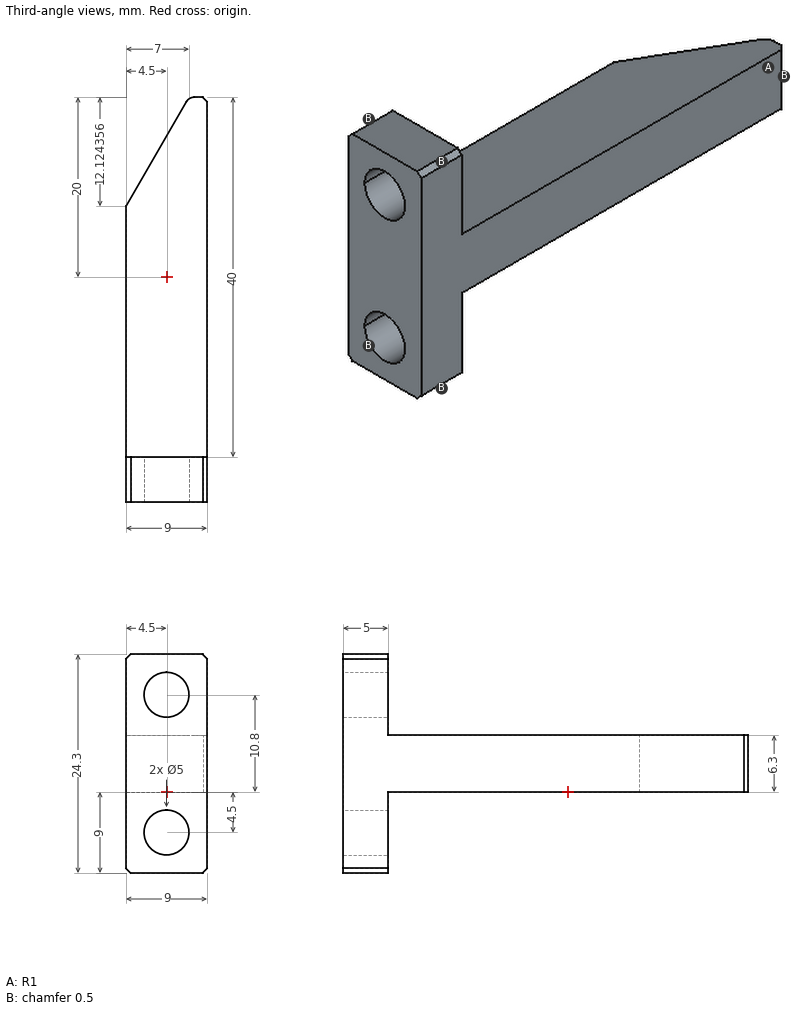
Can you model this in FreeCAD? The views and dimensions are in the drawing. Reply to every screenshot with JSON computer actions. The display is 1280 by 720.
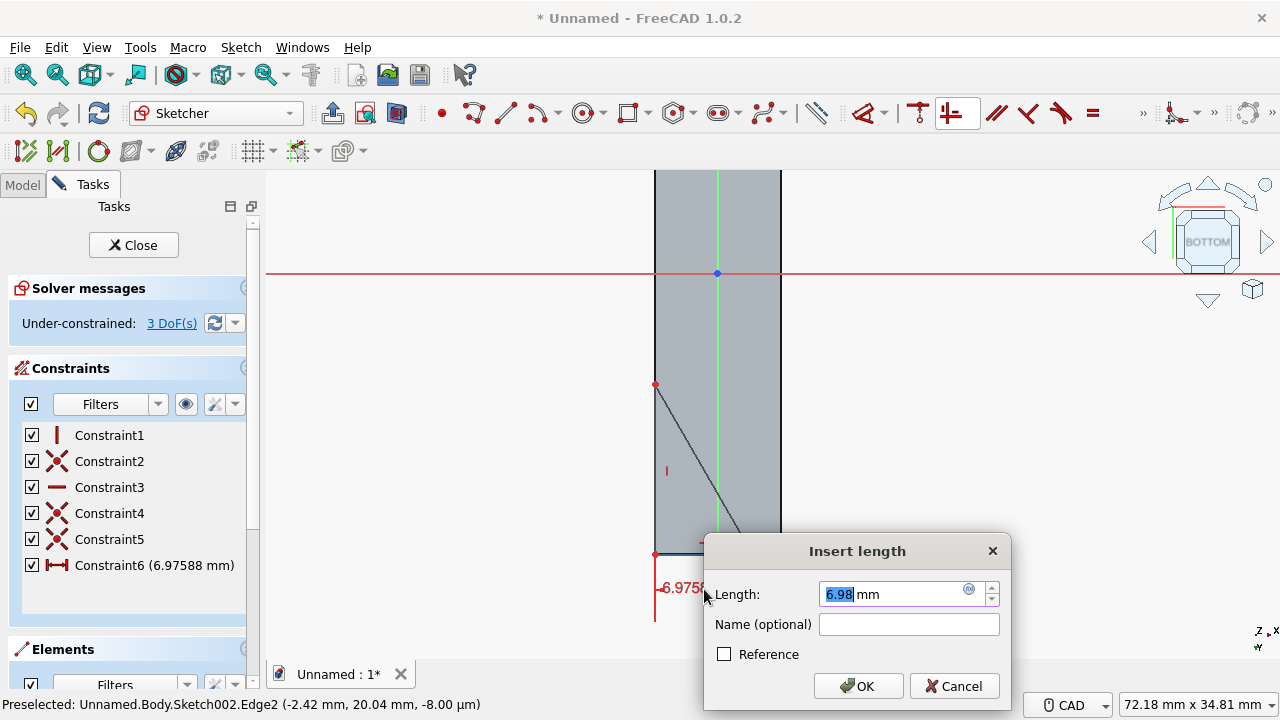
{"action": "type", "text": "7"}
{"action": "key", "text": "Return"}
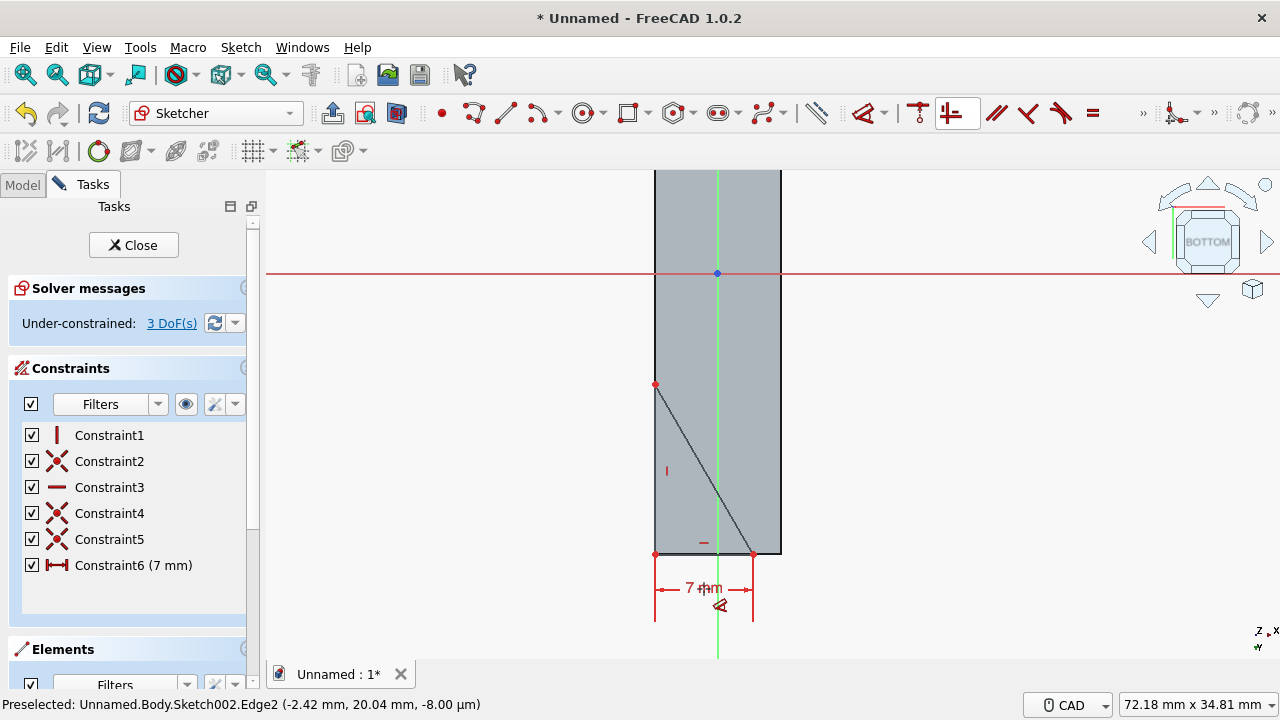
{"action": "left_click", "coordinate": [655, 555]}
{"action": "left_click", "coordinate": [621, 414]}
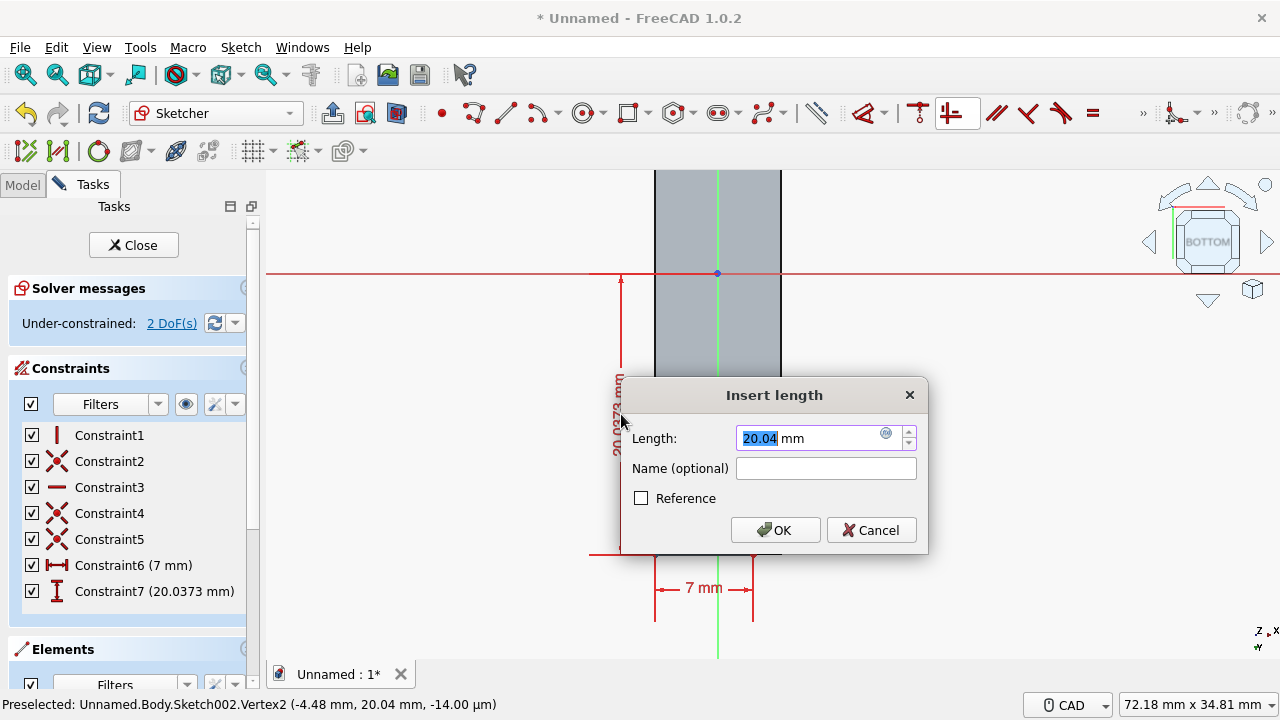
{"action": "type", "text": "20"}
{"action": "key", "text": "Return"}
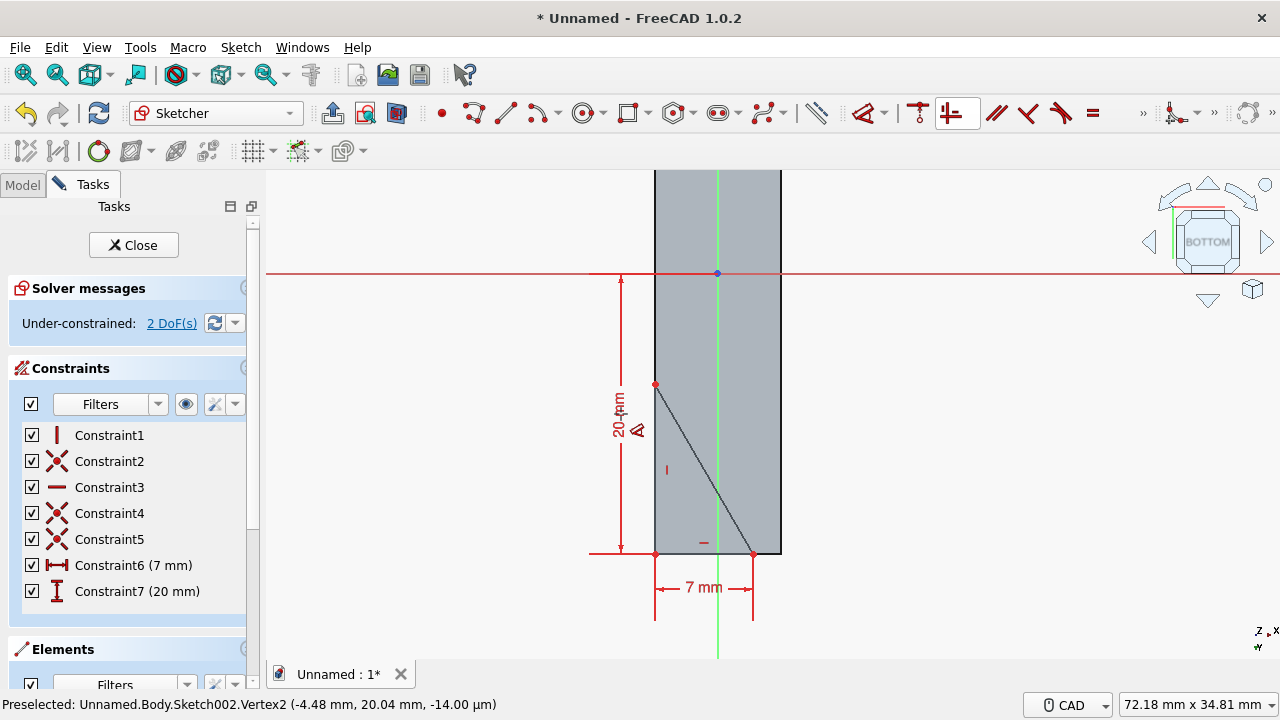
{"action": "left_click", "coordinate": [655, 385]}
{"action": "left_click", "coordinate": [686, 240]}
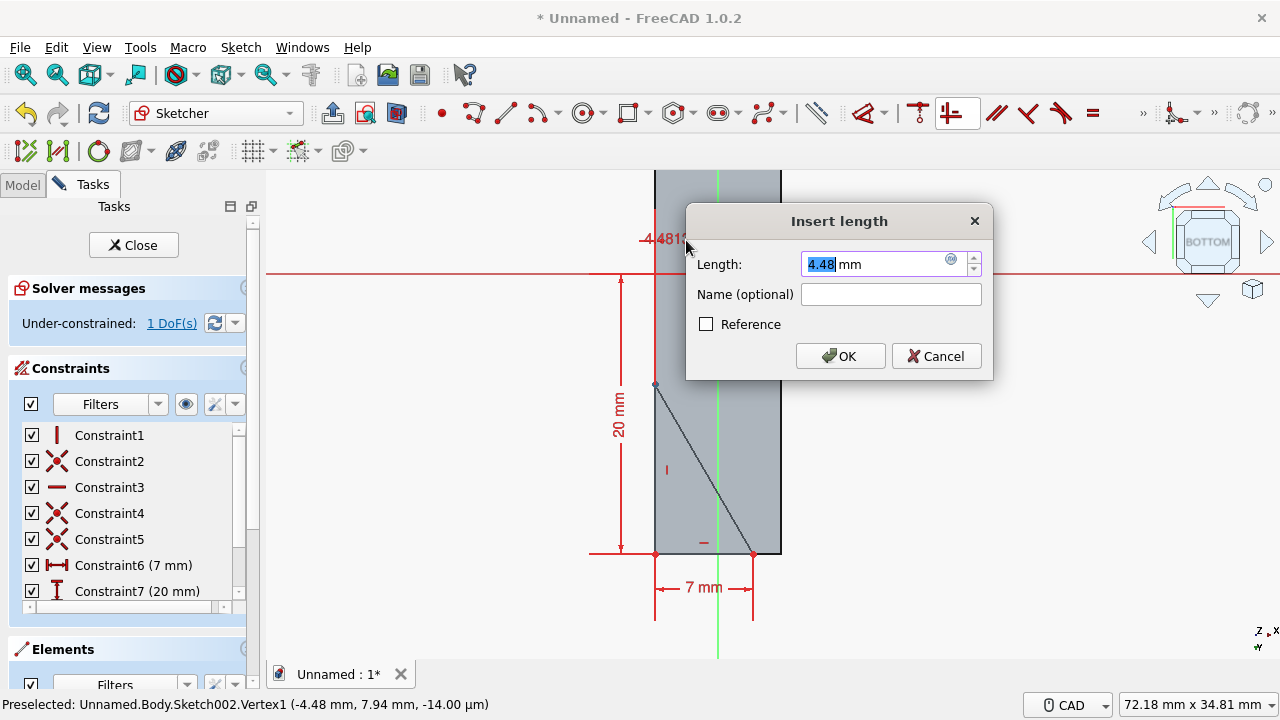
{"action": "type", "text": "4.5"}
{"action": "key", "text": "Return"}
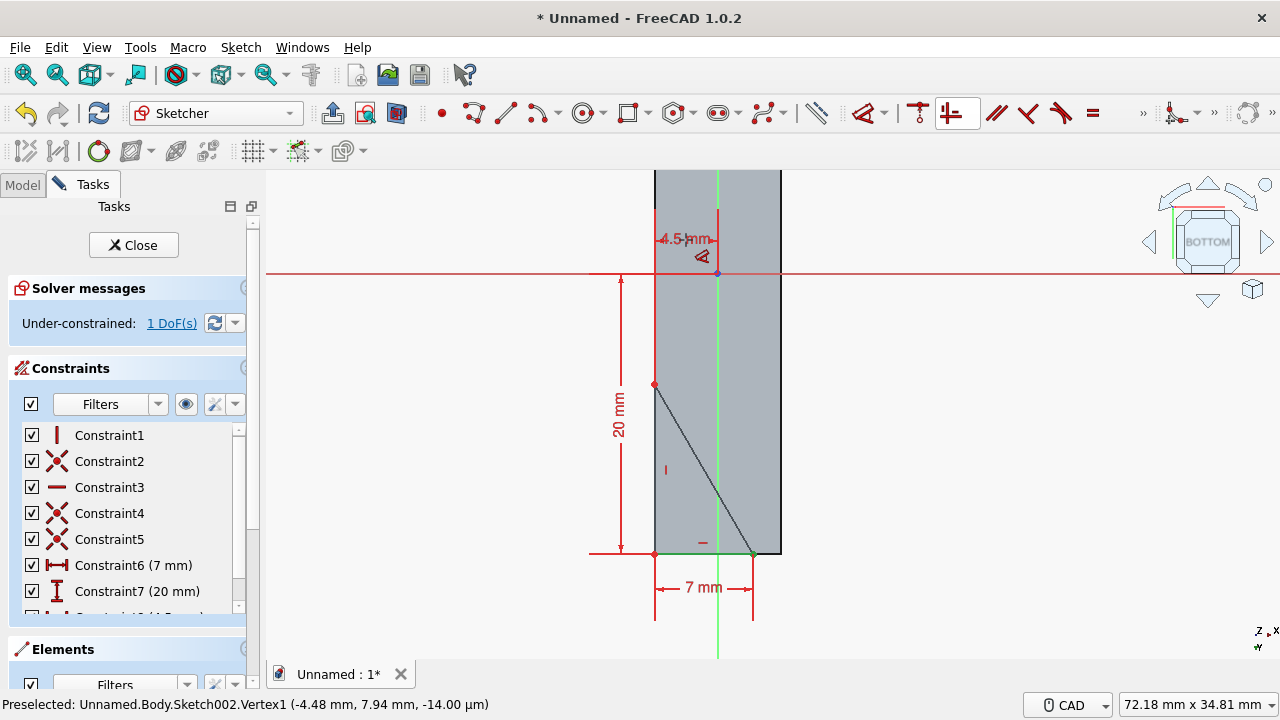
{"action": "left_click", "coordinate": [655, 436]}
{"action": "left_click", "coordinate": [621, 470]}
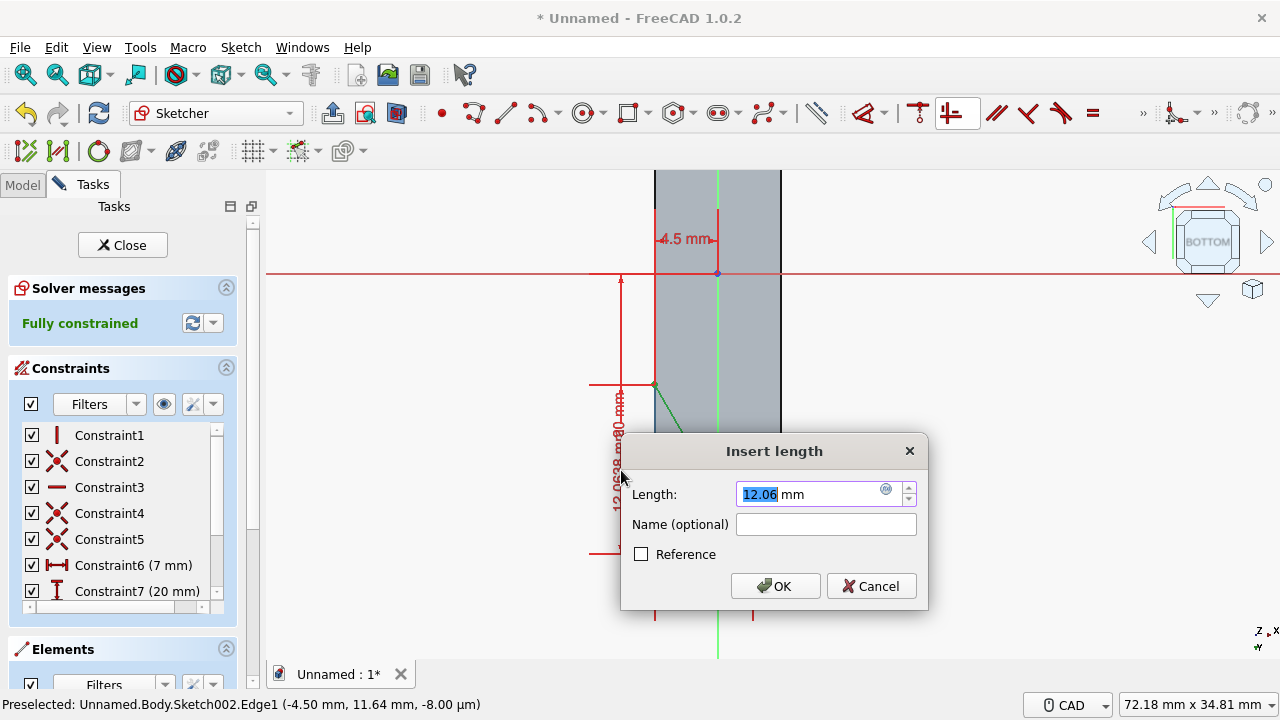
{"action": "type", "text": "12.124356"}
{"action": "key", "text": "Return"}
{"action": "key", "text": "Escape"}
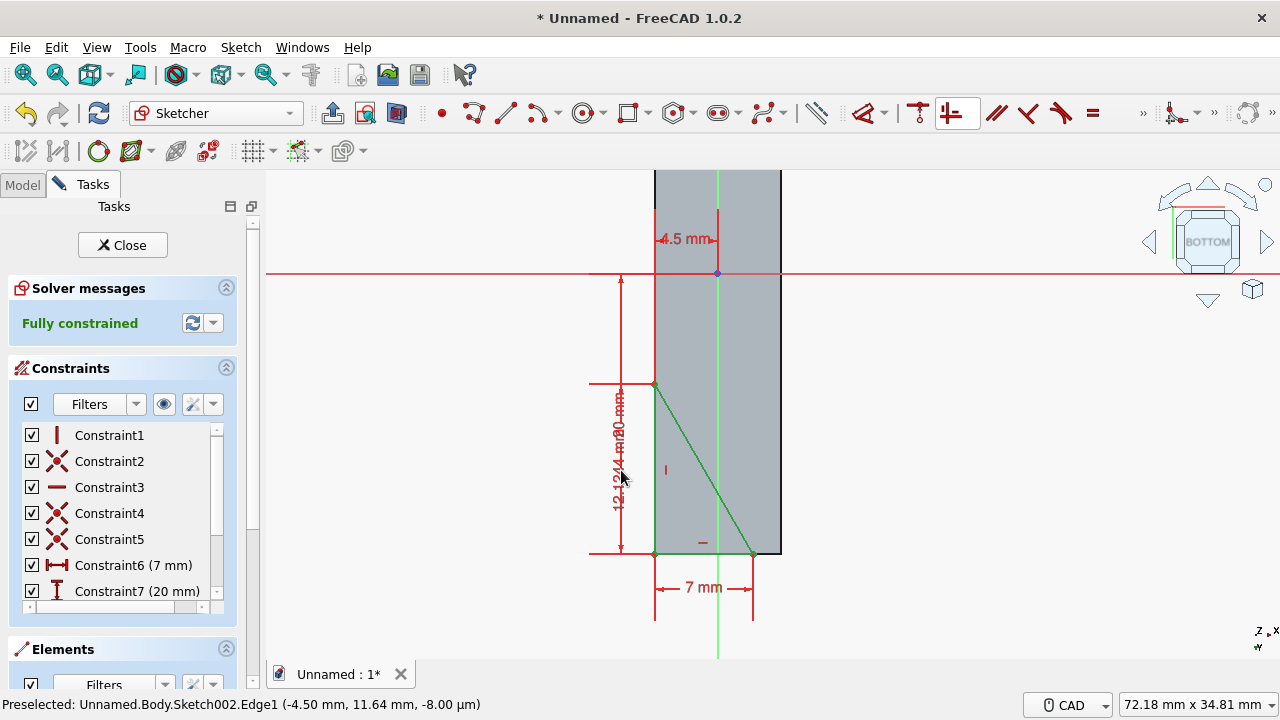
{"action": "left_click", "coordinate": [123, 245]}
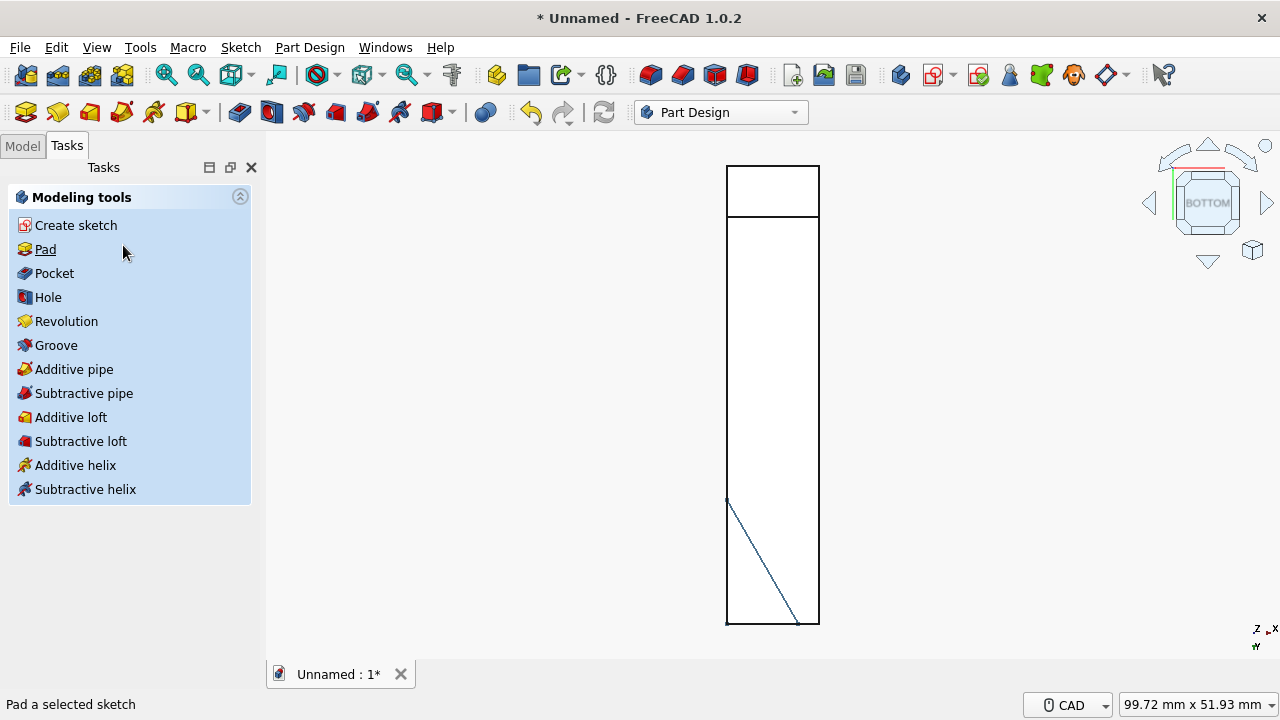
{"action": "left_click", "coordinate": [240, 112]}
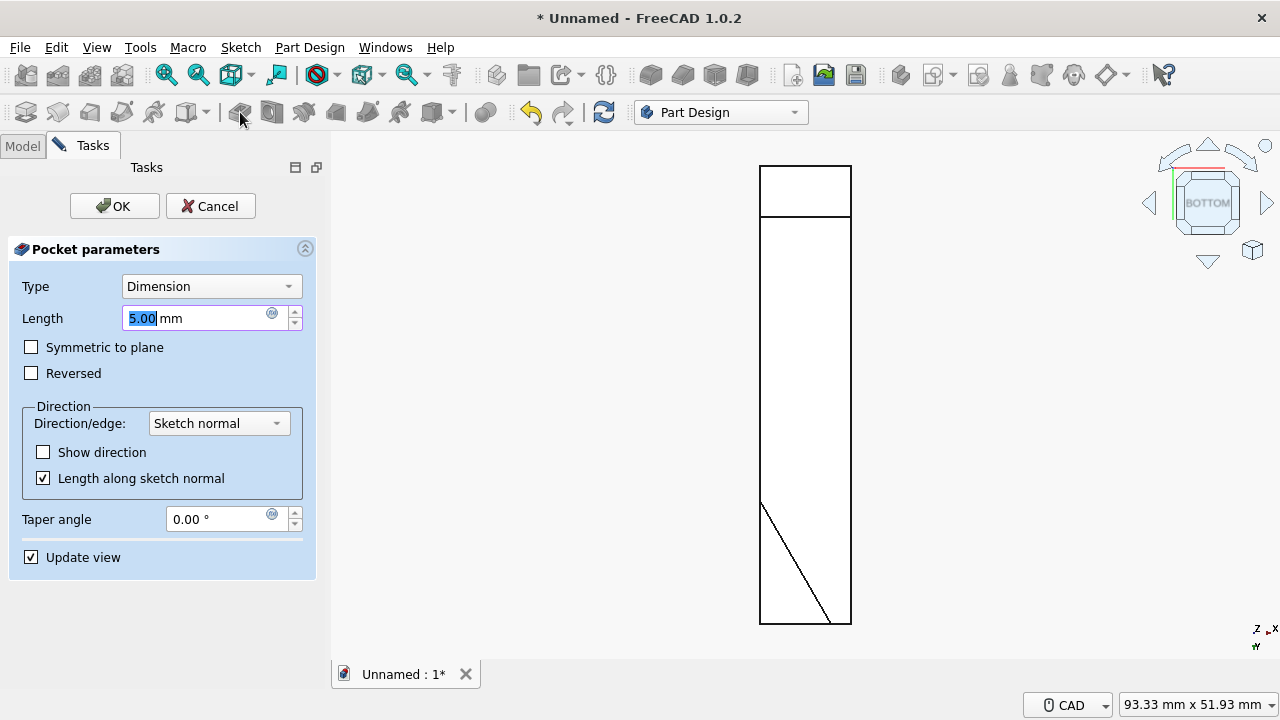
{"action": "left_click", "coordinate": [212, 286]}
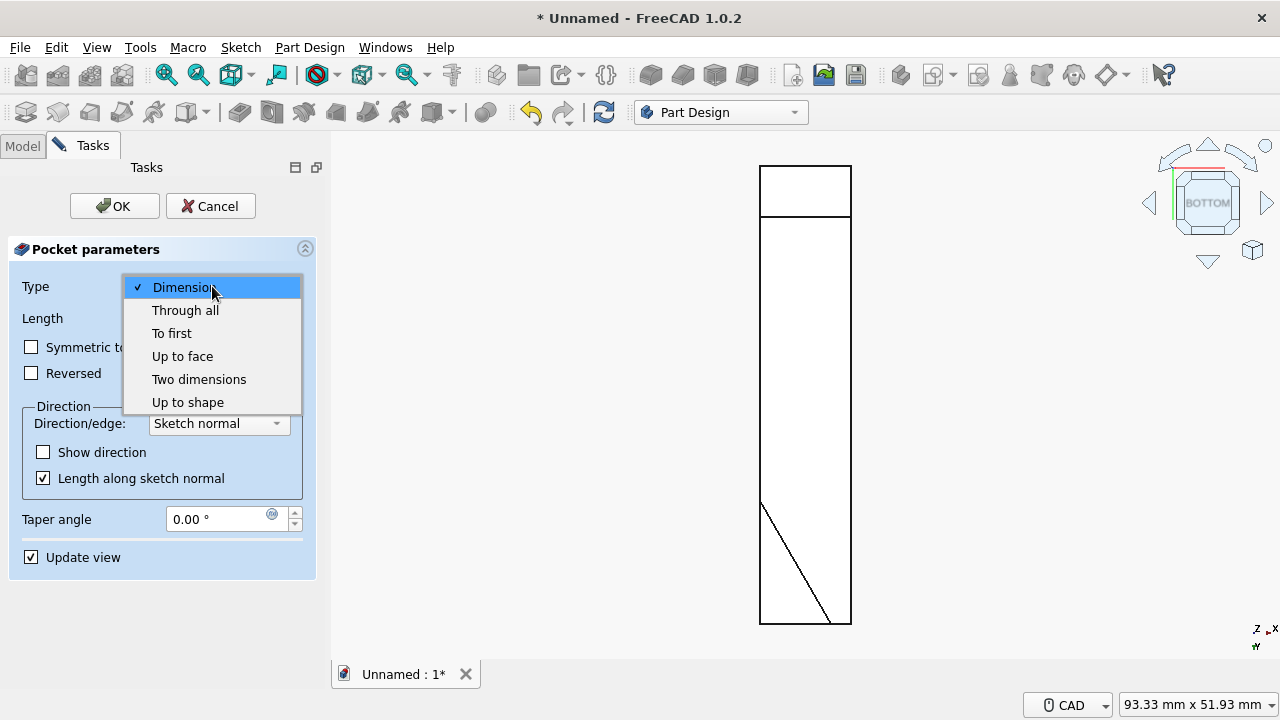
{"action": "left_click", "coordinate": [212, 310]}